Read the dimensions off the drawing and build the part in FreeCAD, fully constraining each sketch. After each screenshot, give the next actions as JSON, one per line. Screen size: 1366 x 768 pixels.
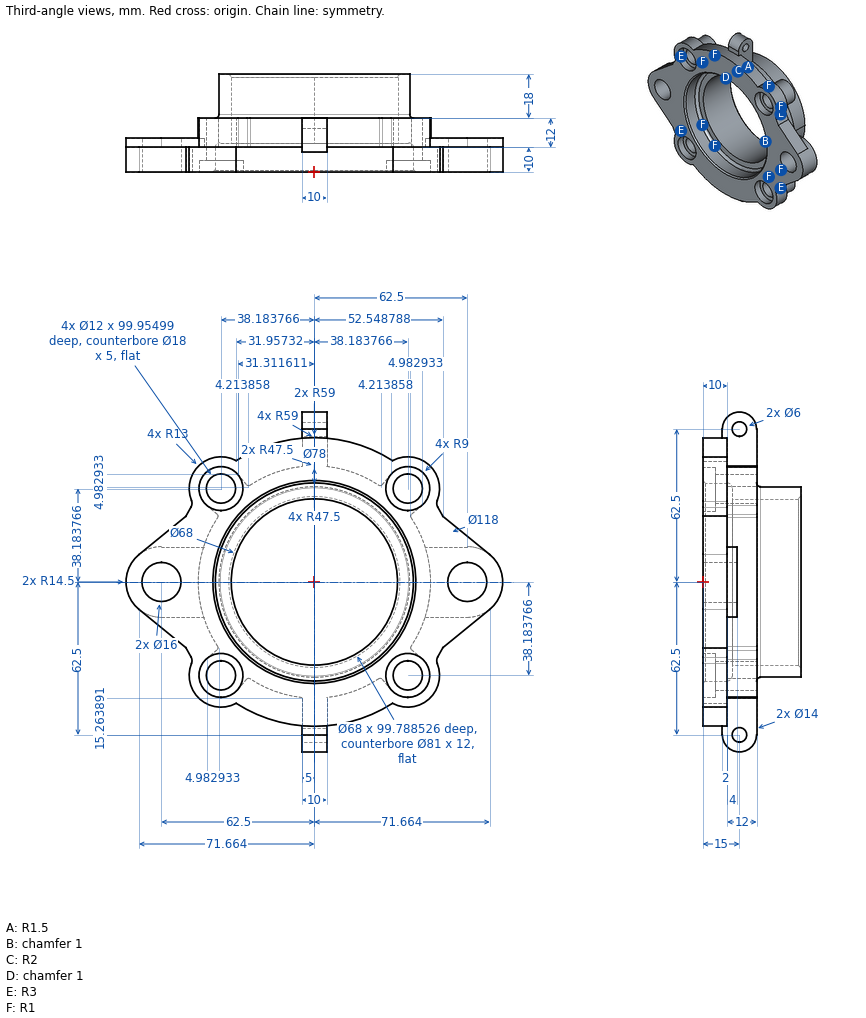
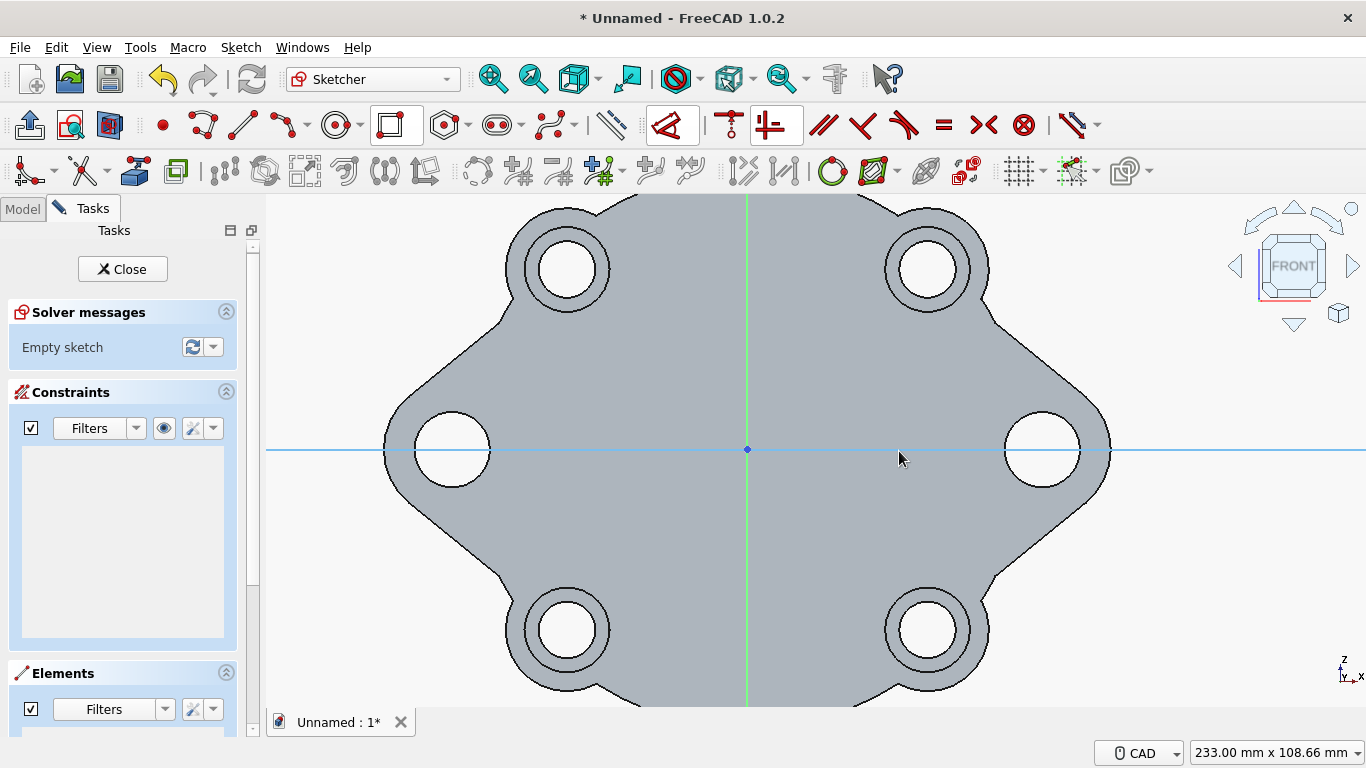
{"action": "left_click", "coordinate": [336, 126]}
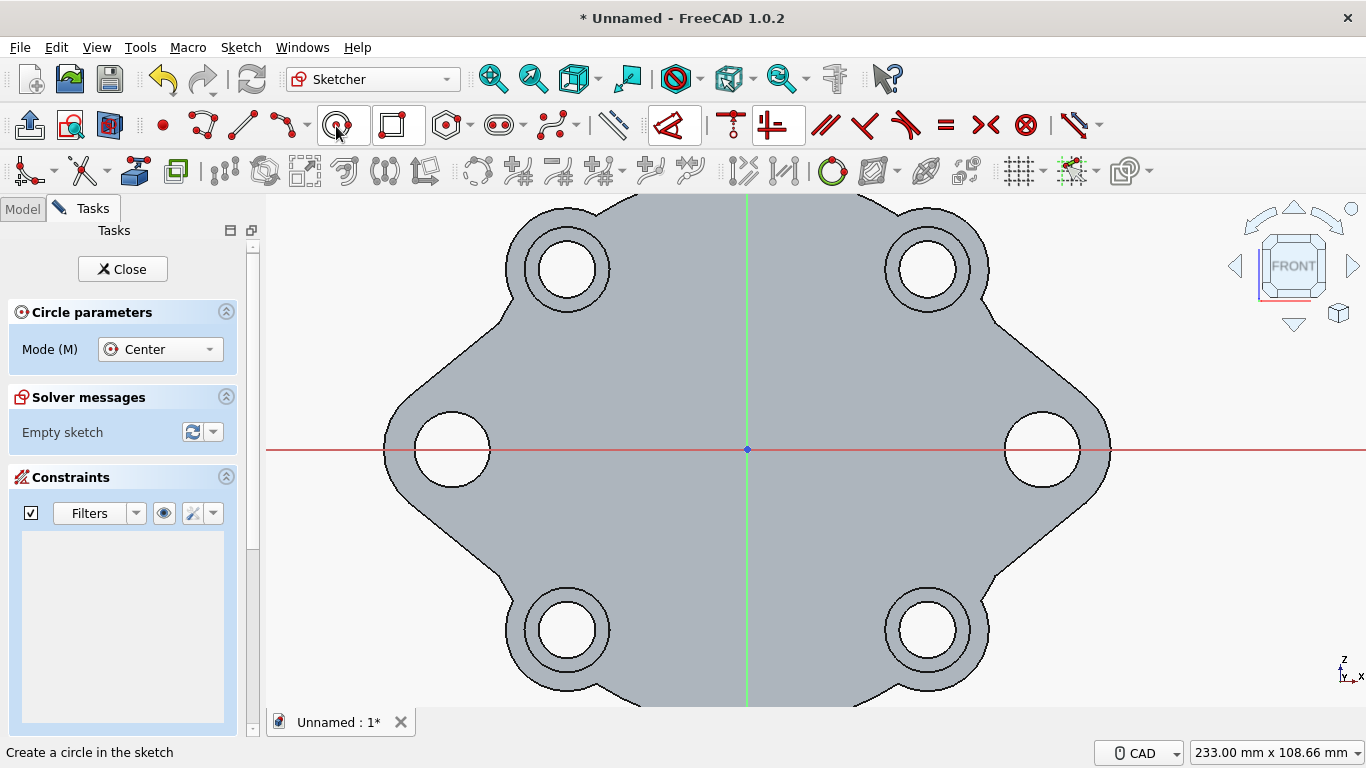
{"action": "left_click", "coordinate": [747, 450]}
{"action": "left_click", "coordinate": [861, 336]}
{"action": "key", "text": "Escape"}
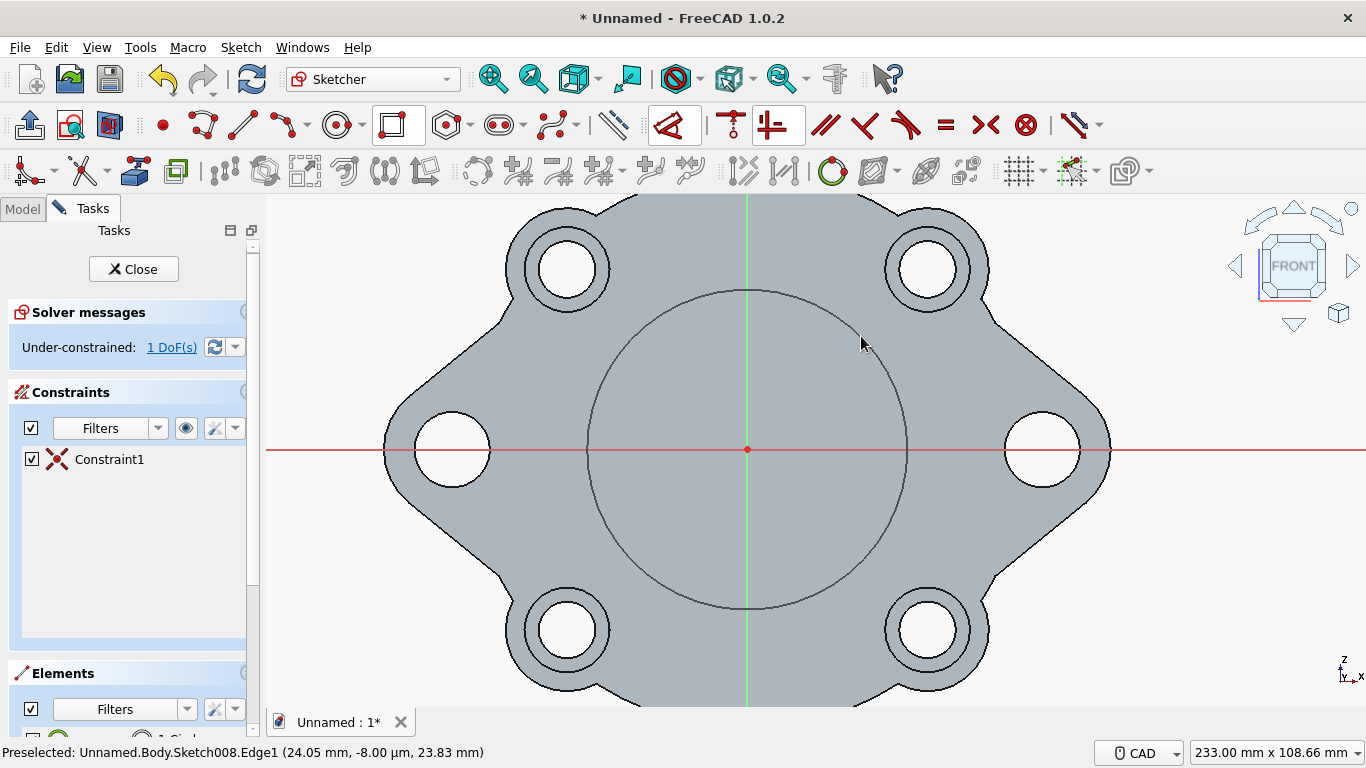
{"action": "left_click", "coordinate": [860, 336]}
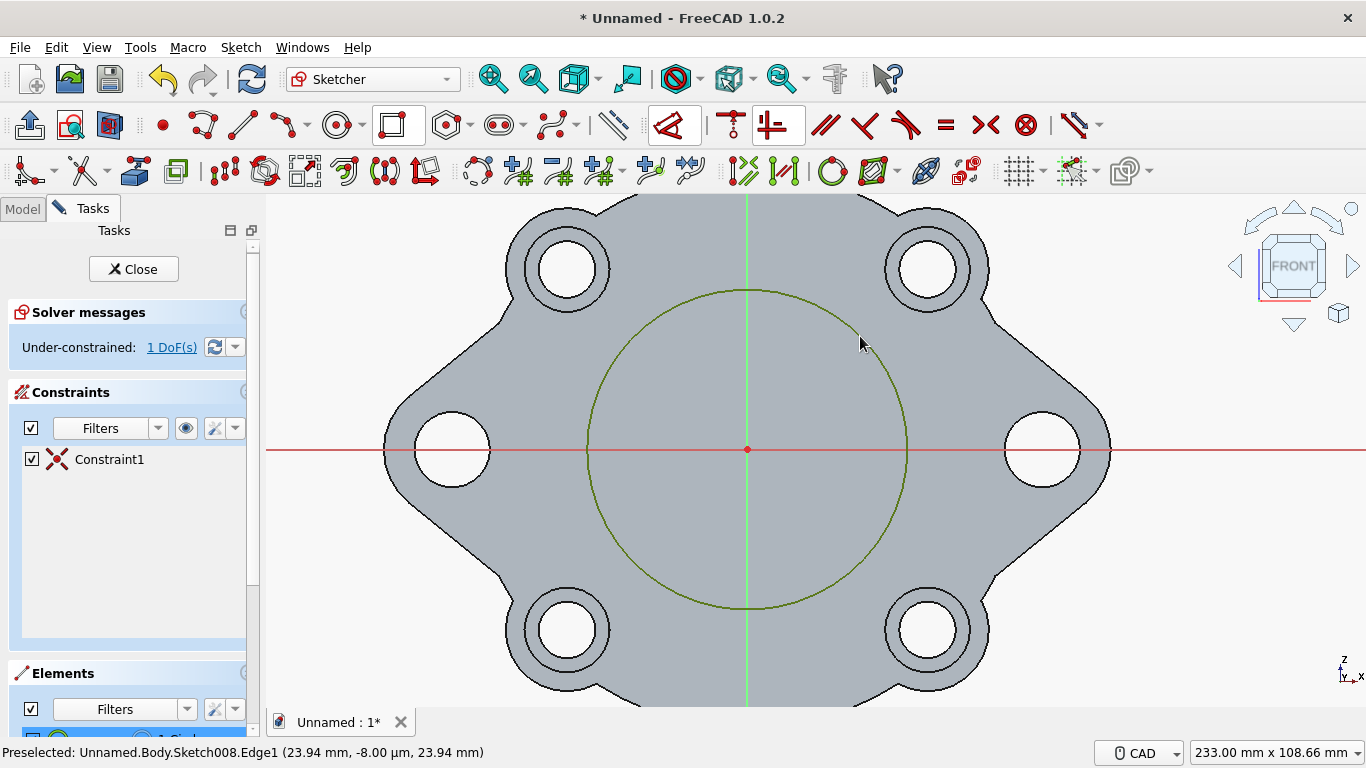
{"action": "key", "text": "k o"}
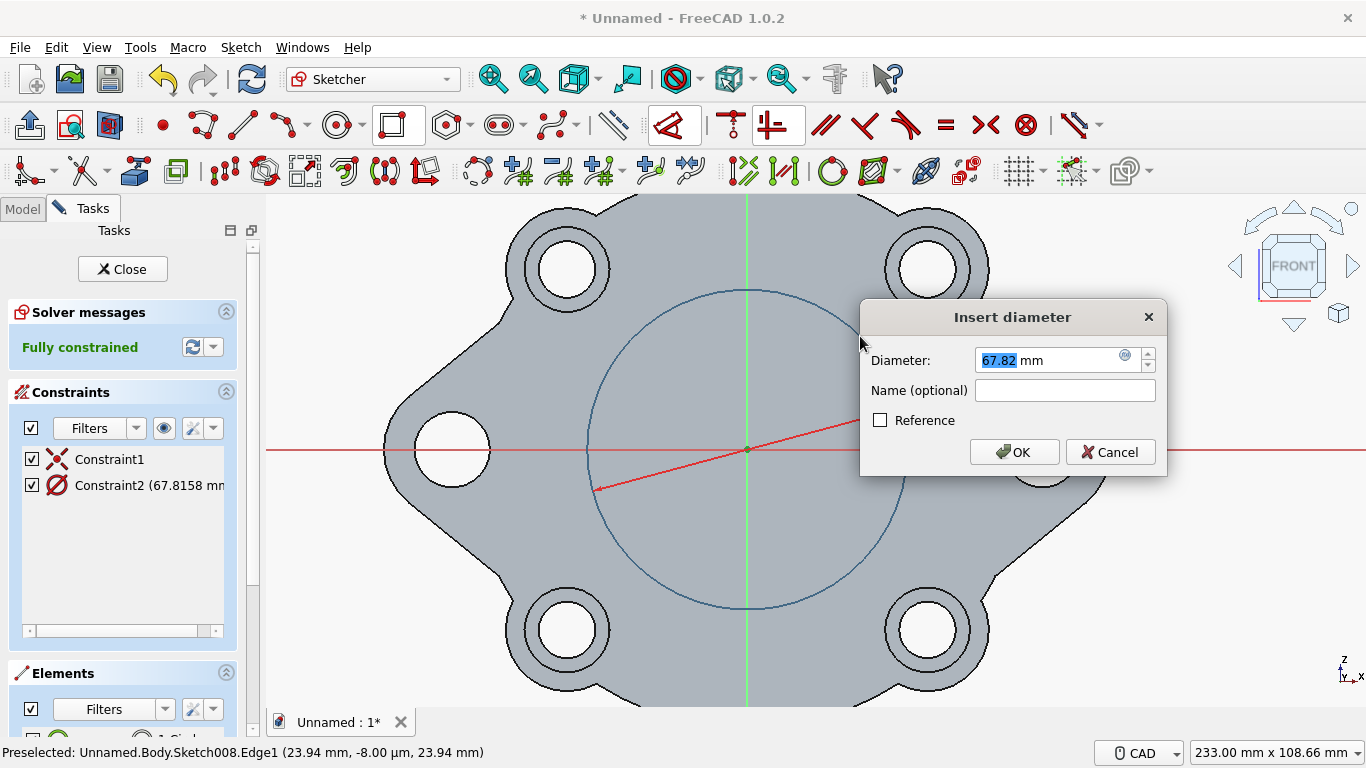
{"action": "type", "text": "68"}
{"action": "key", "text": "Return"}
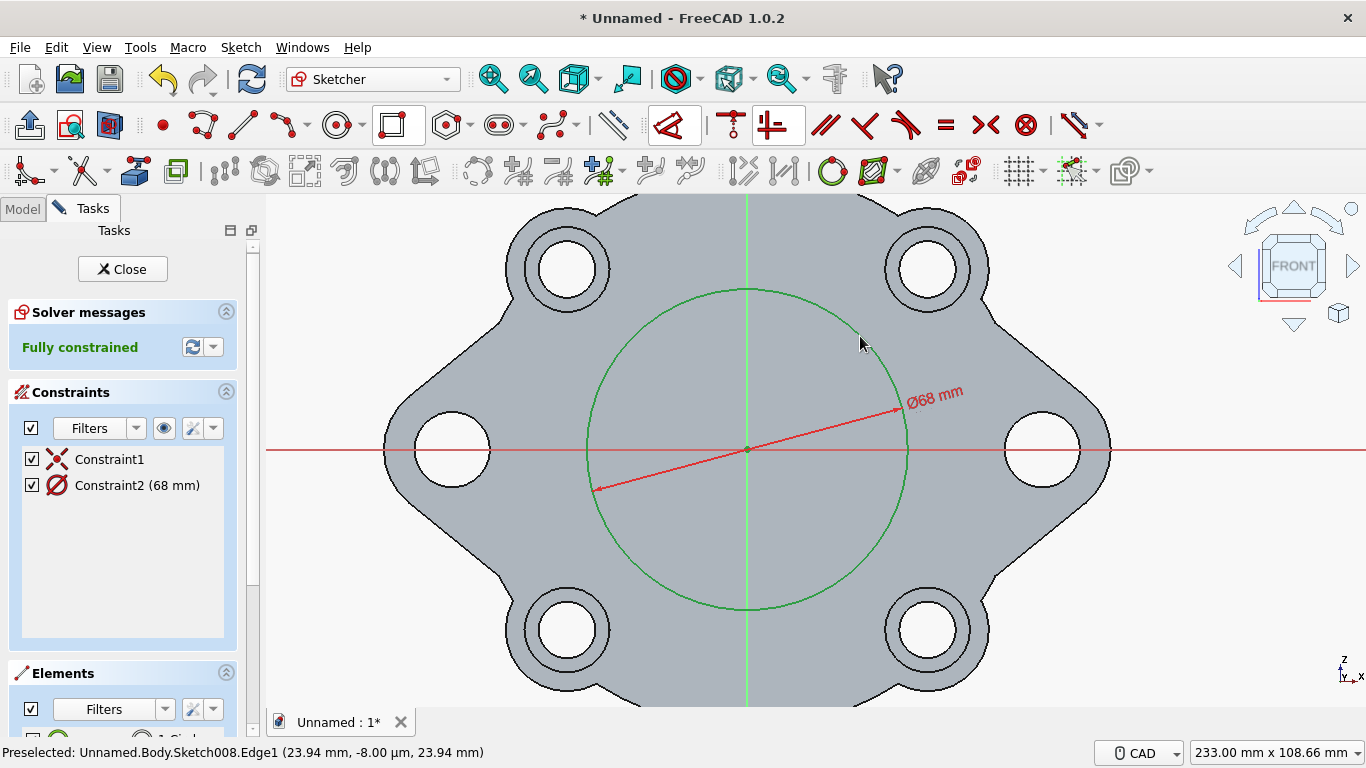
{"action": "left_click", "coordinate": [123, 269]}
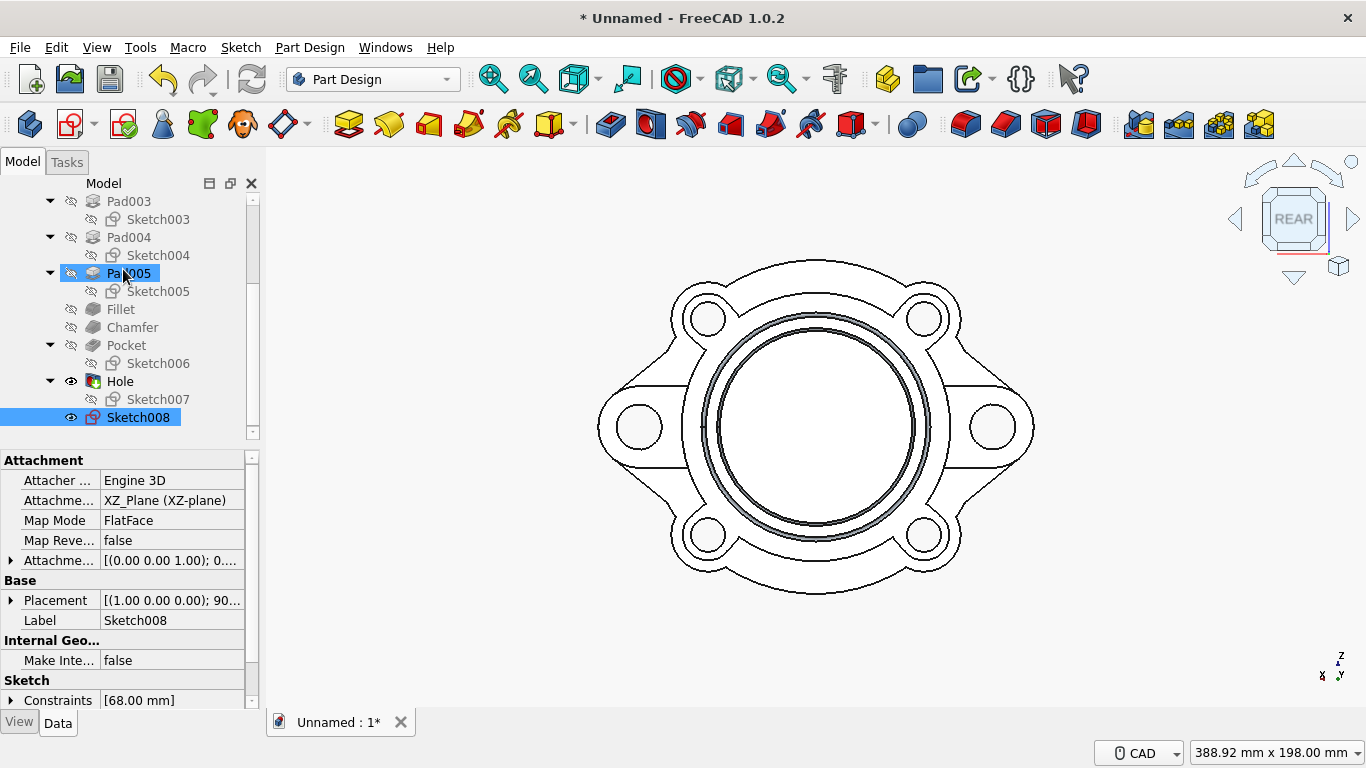
{"action": "left_click", "coordinate": [652, 124]}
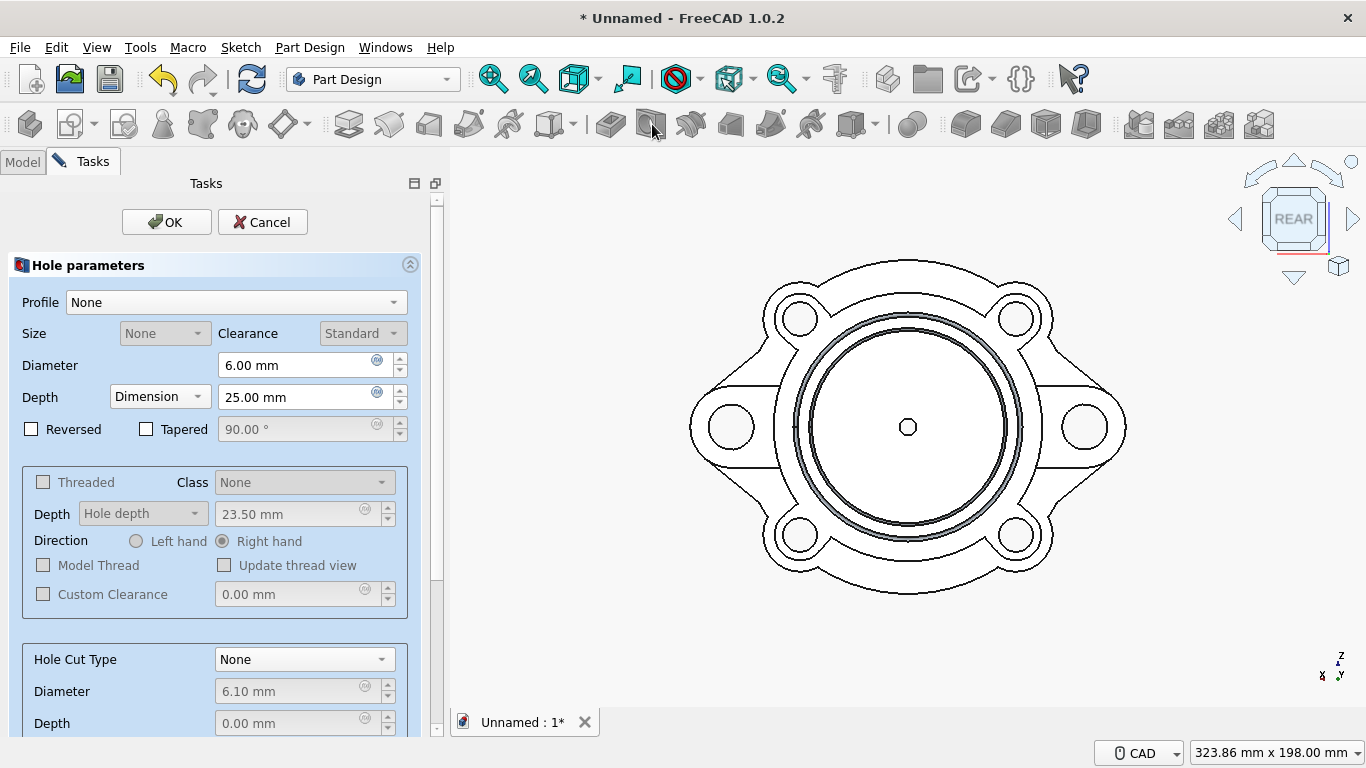
{"action": "triple_click", "coordinate": [305, 365]}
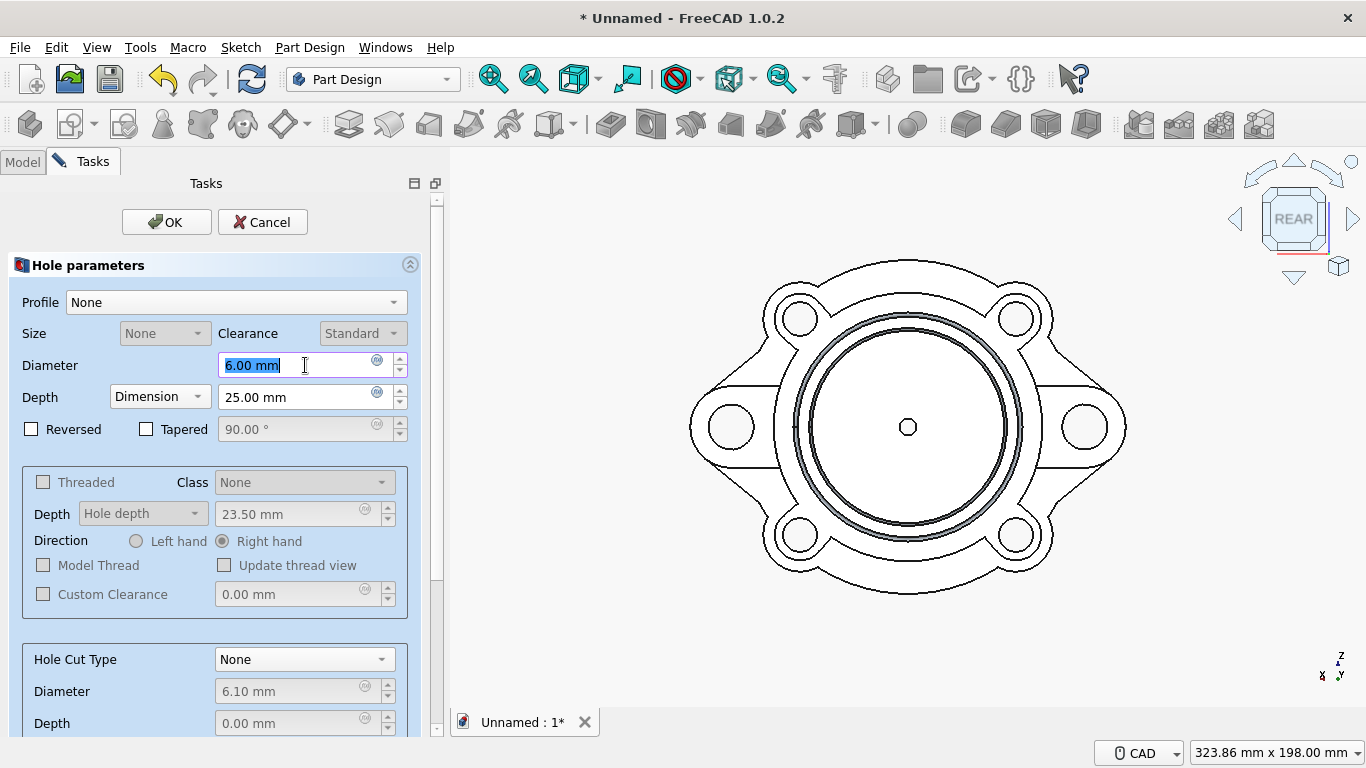
{"action": "type", "text": "68"}
{"action": "key", "text": "Tab"}